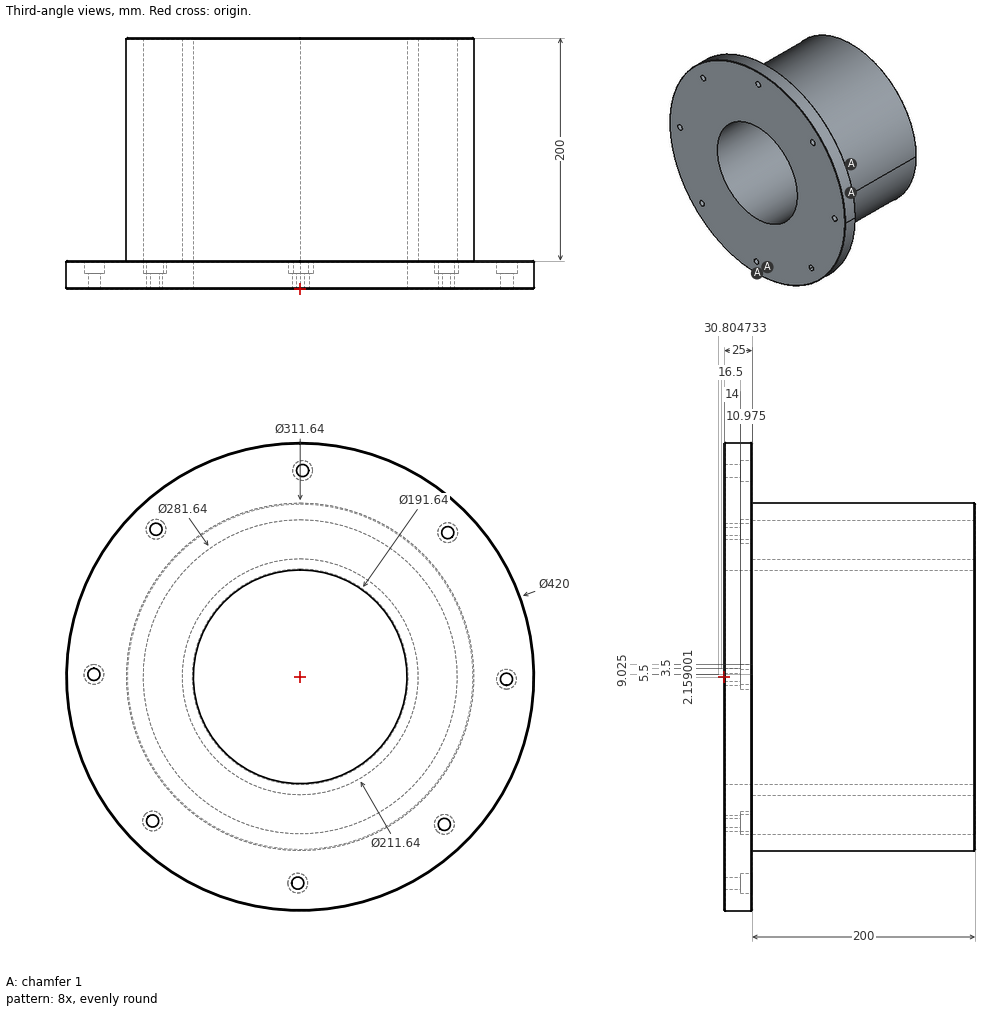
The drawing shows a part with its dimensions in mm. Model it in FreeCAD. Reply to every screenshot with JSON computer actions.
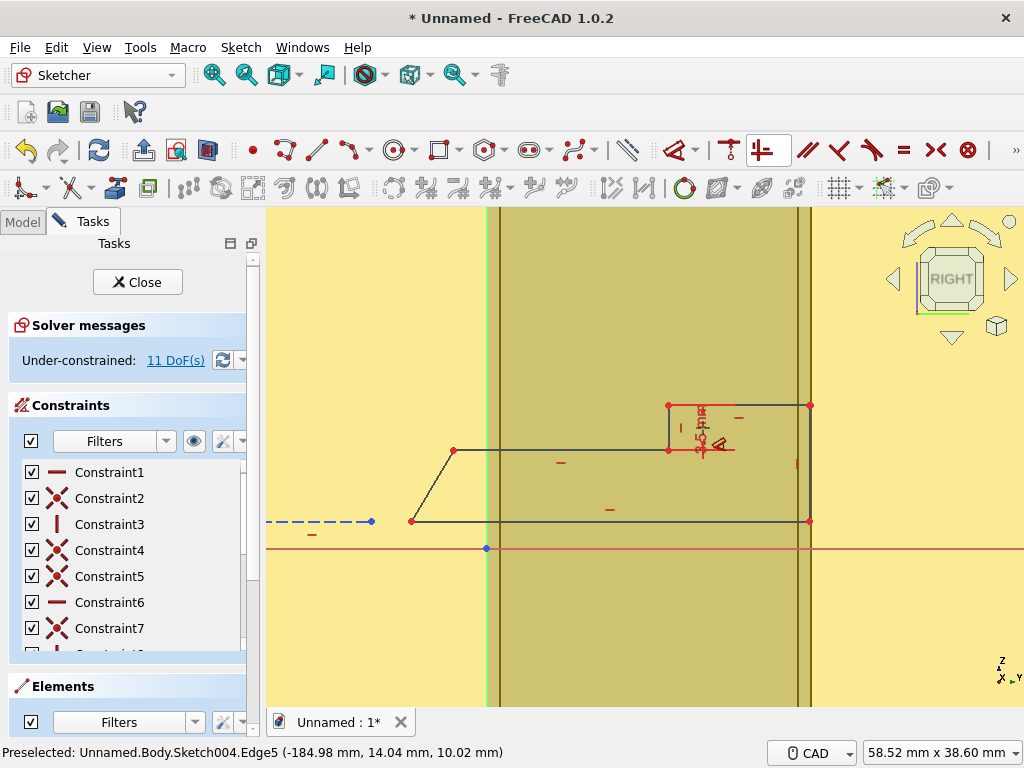
{"action": "left_click", "coordinate": [810, 522]}
{"action": "left_click", "coordinate": [648, 583]}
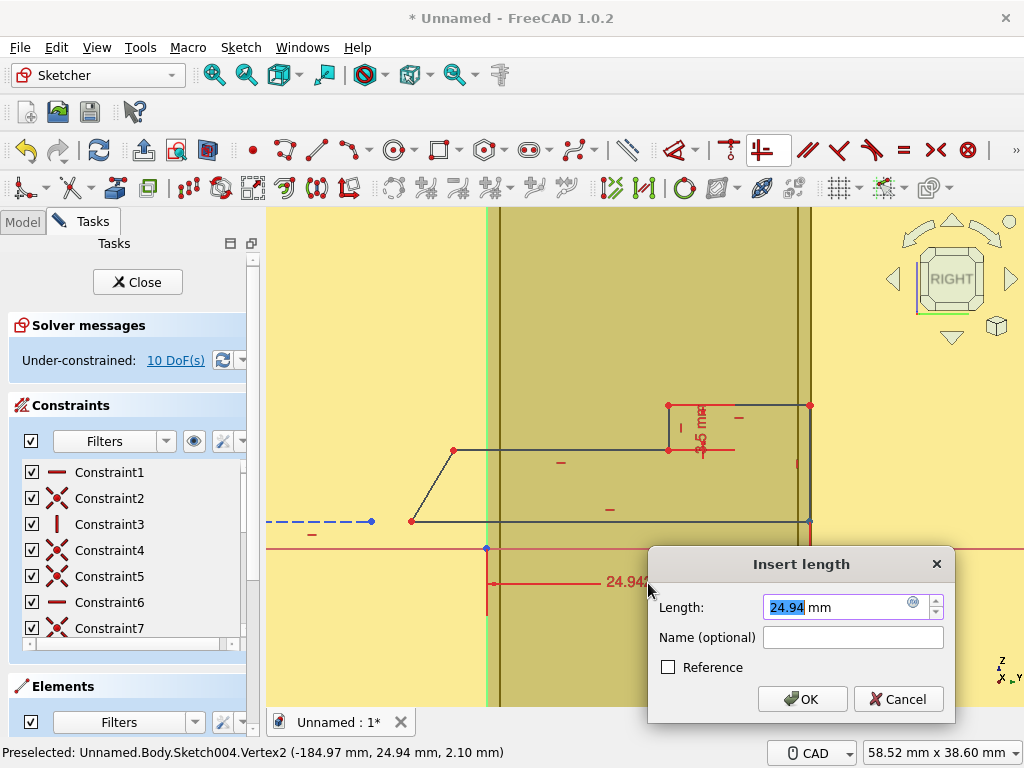
{"action": "type", "text": "25"}
{"action": "key", "text": "Return"}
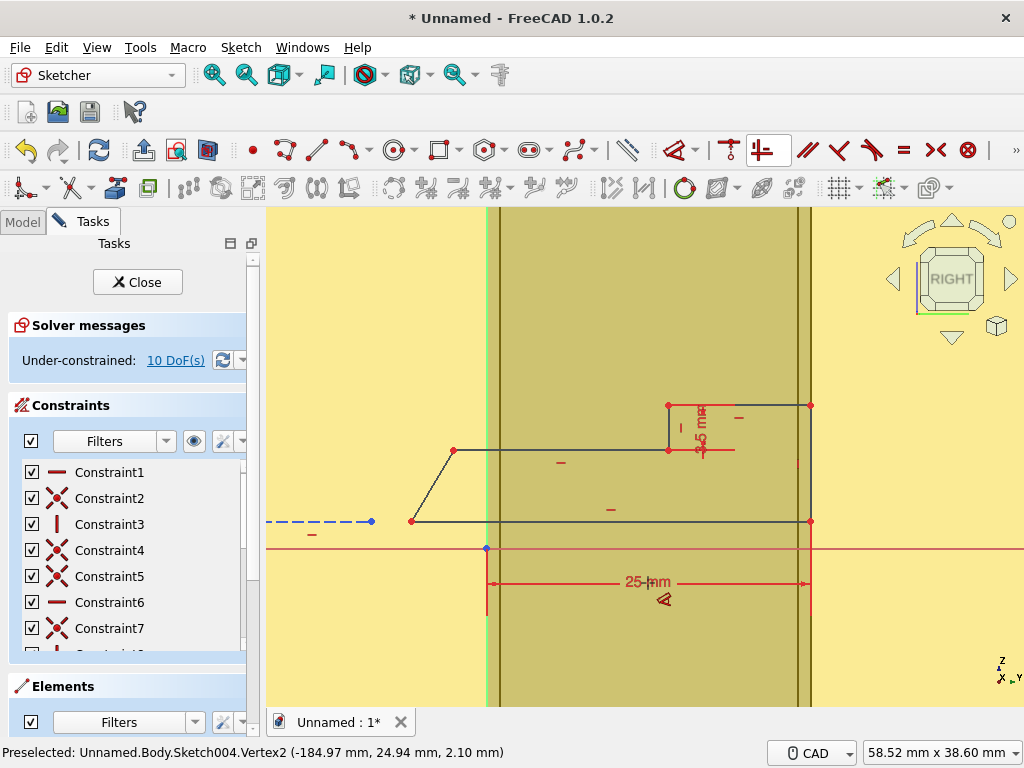
{"action": "left_click", "coordinate": [669, 405]}
{"action": "left_click", "coordinate": [578, 583]}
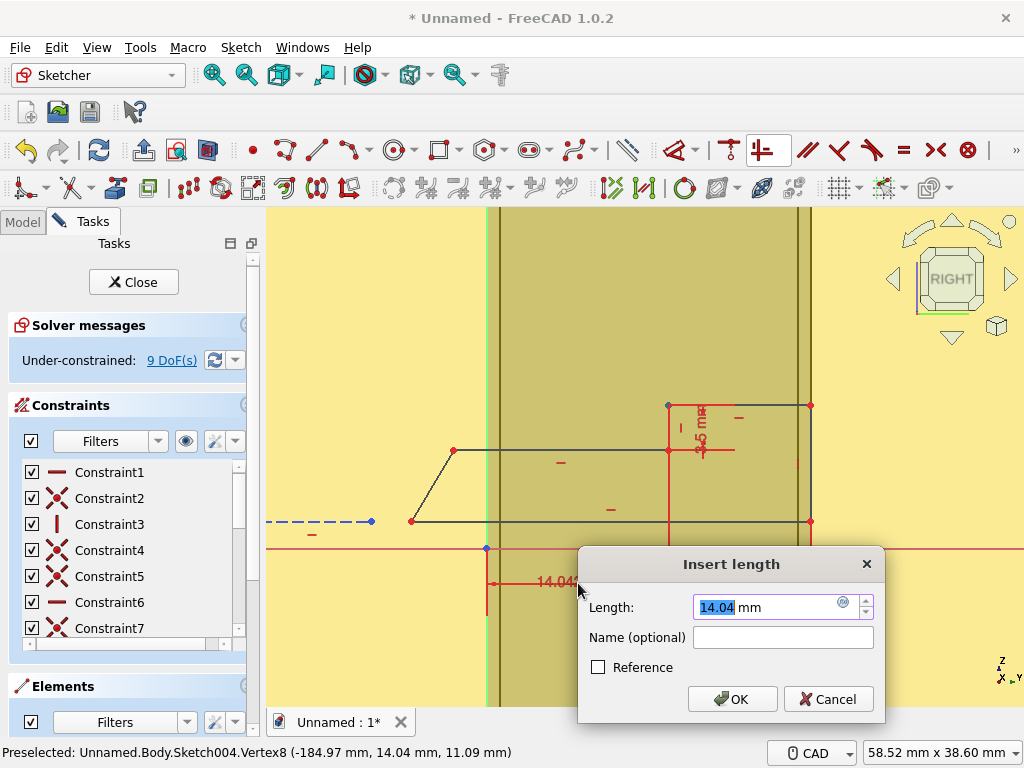
{"action": "type", "text": "14"}
{"action": "key", "text": "Return"}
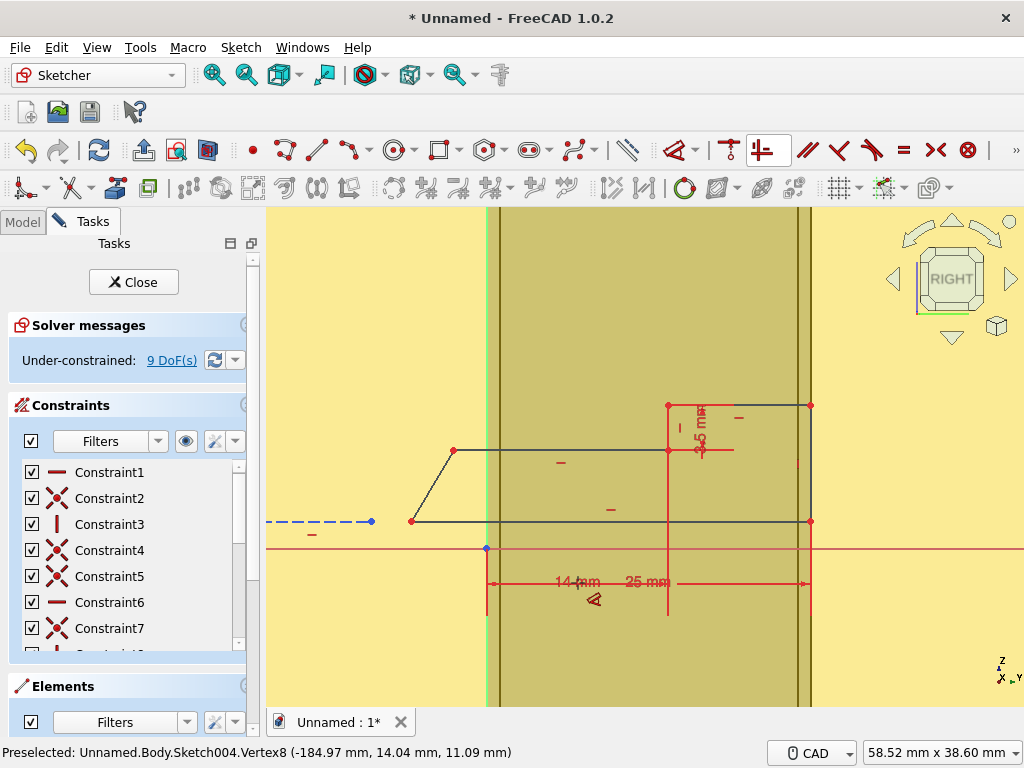
{"action": "left_click", "coordinate": [604, 450]}
{"action": "left_click", "coordinate": [561, 416]}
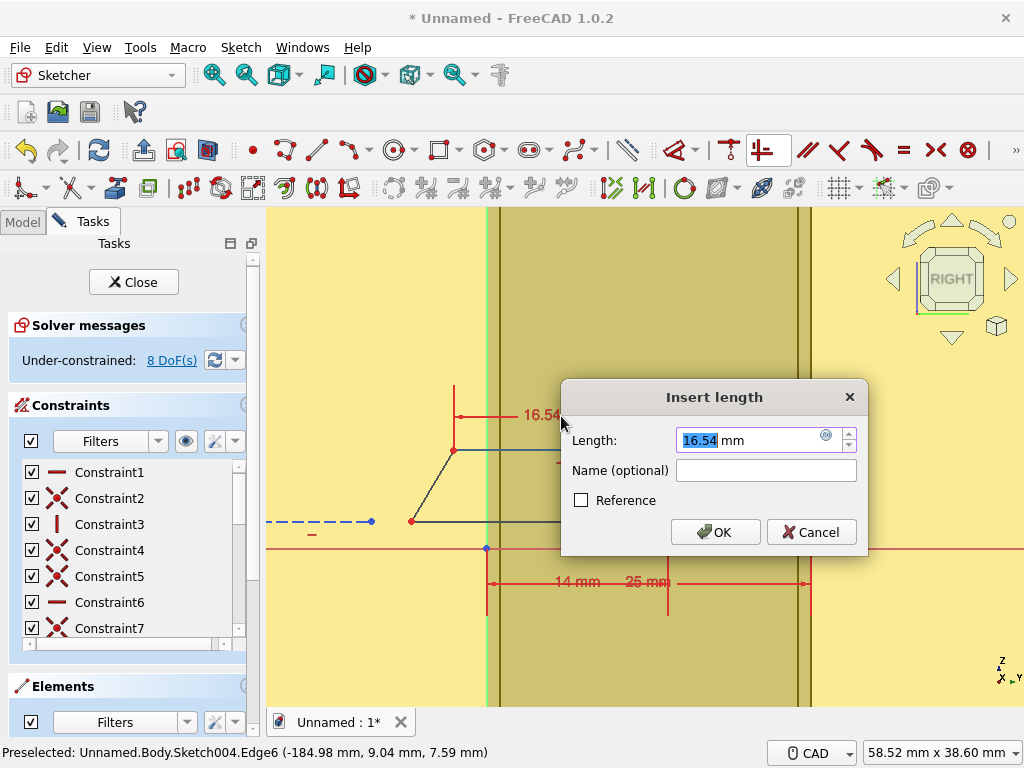
{"action": "type", "text": "16.5"}
{"action": "key", "text": "Return"}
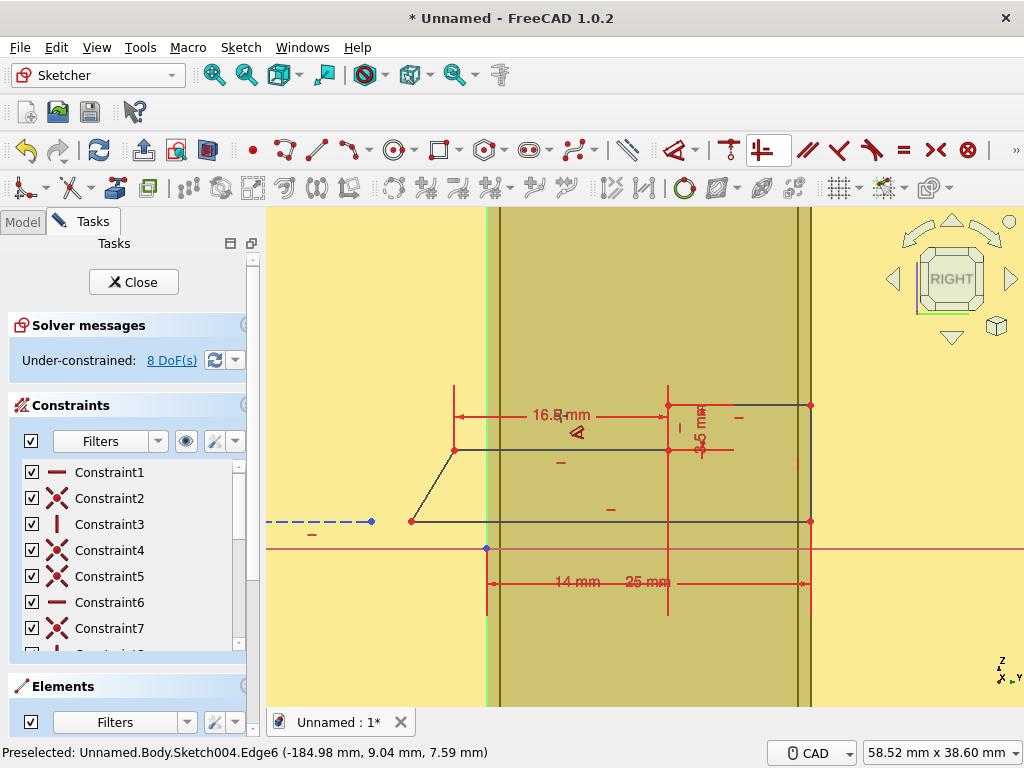
{"action": "left_click", "coordinate": [442, 472]}
{"action": "left_click", "coordinate": [378, 486]}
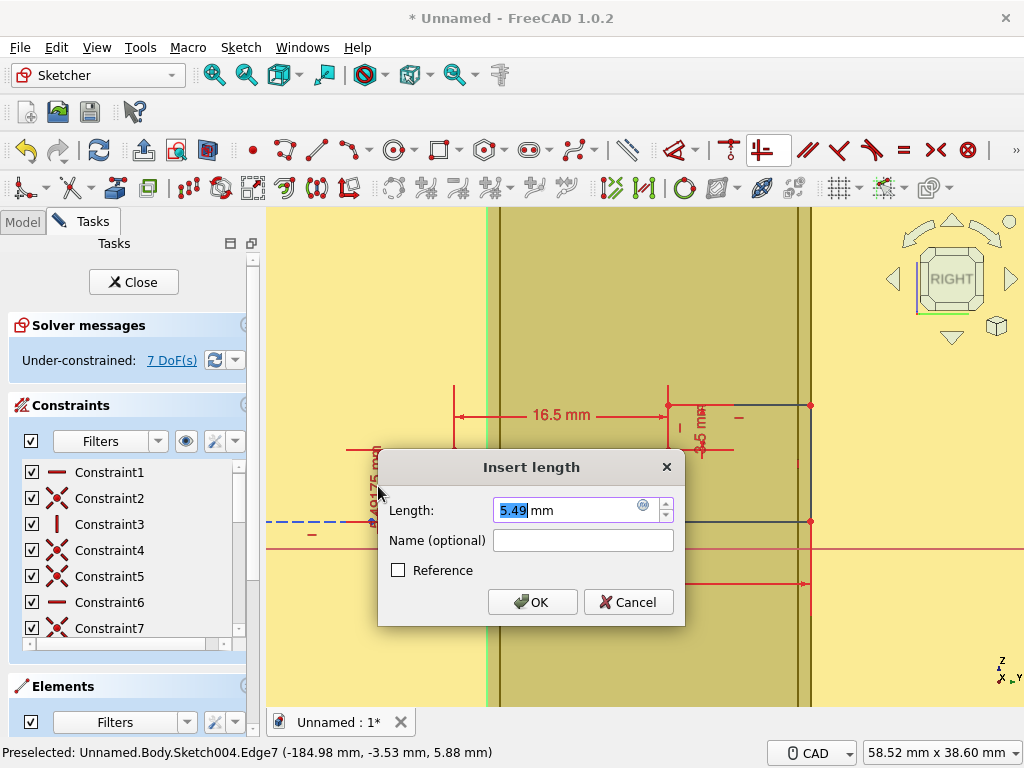
{"action": "type", "text": "5.5"}
{"action": "key", "text": "Return"}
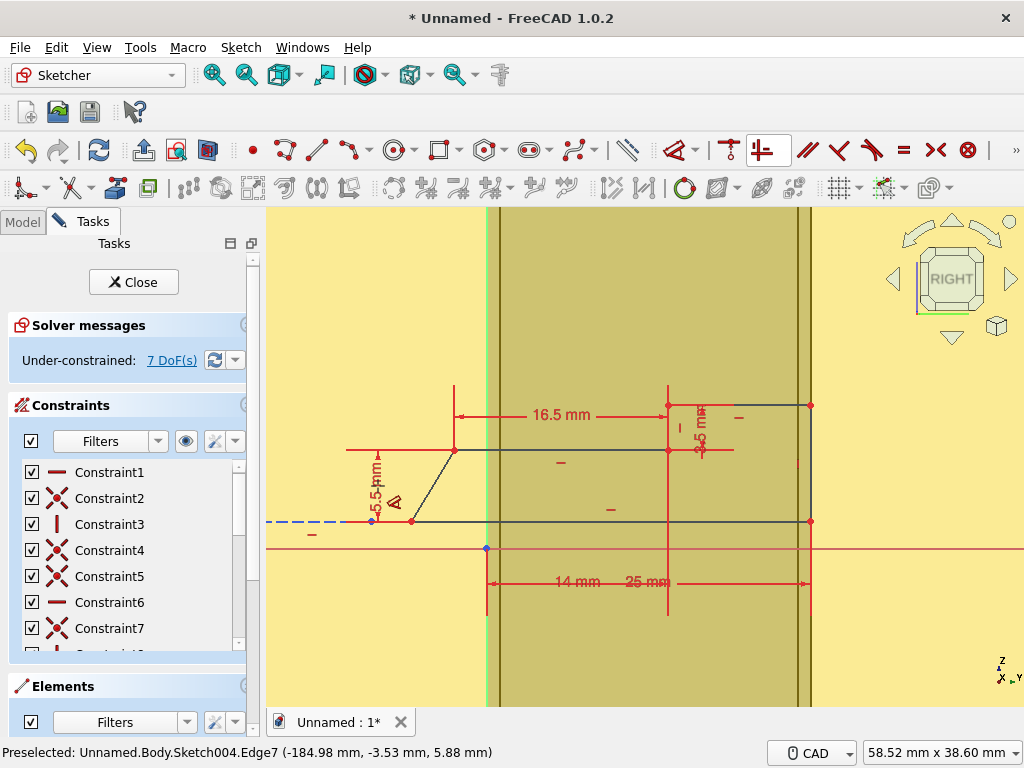
{"action": "left_click", "coordinate": [811, 487]}
{"action": "left_click", "coordinate": [845, 463]}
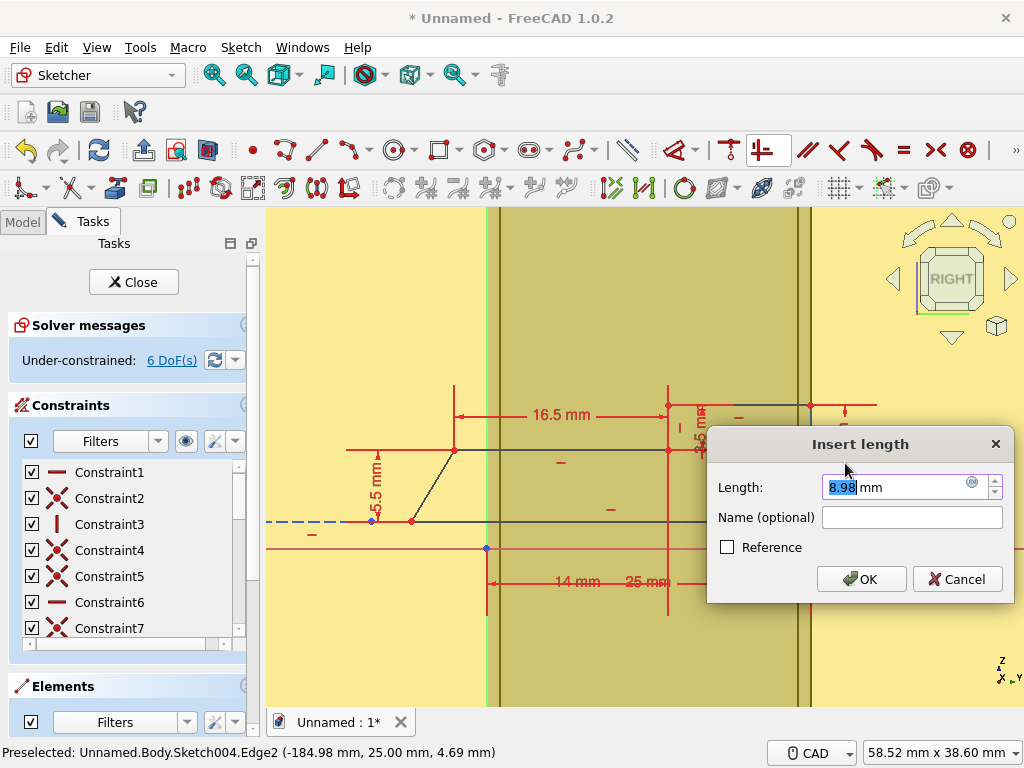
{"action": "type", "text": "9.025"}
{"action": "key", "text": "Return"}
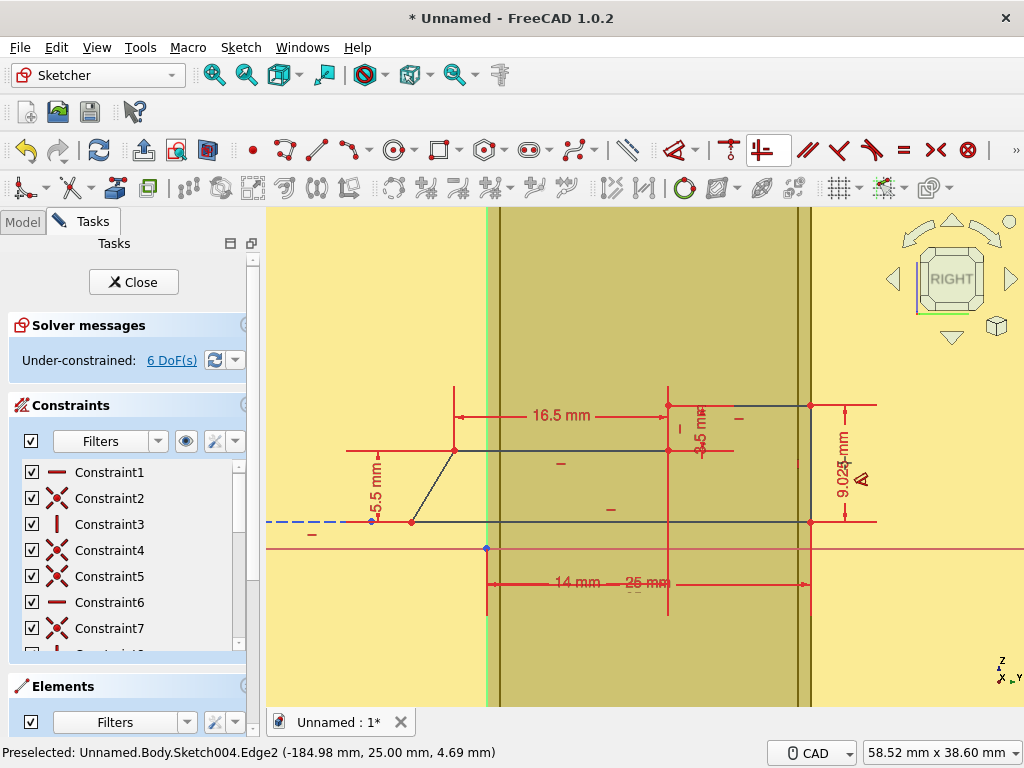
{"action": "left_click", "coordinate": [768, 406]}
{"action": "left_click", "coordinate": [739, 372]}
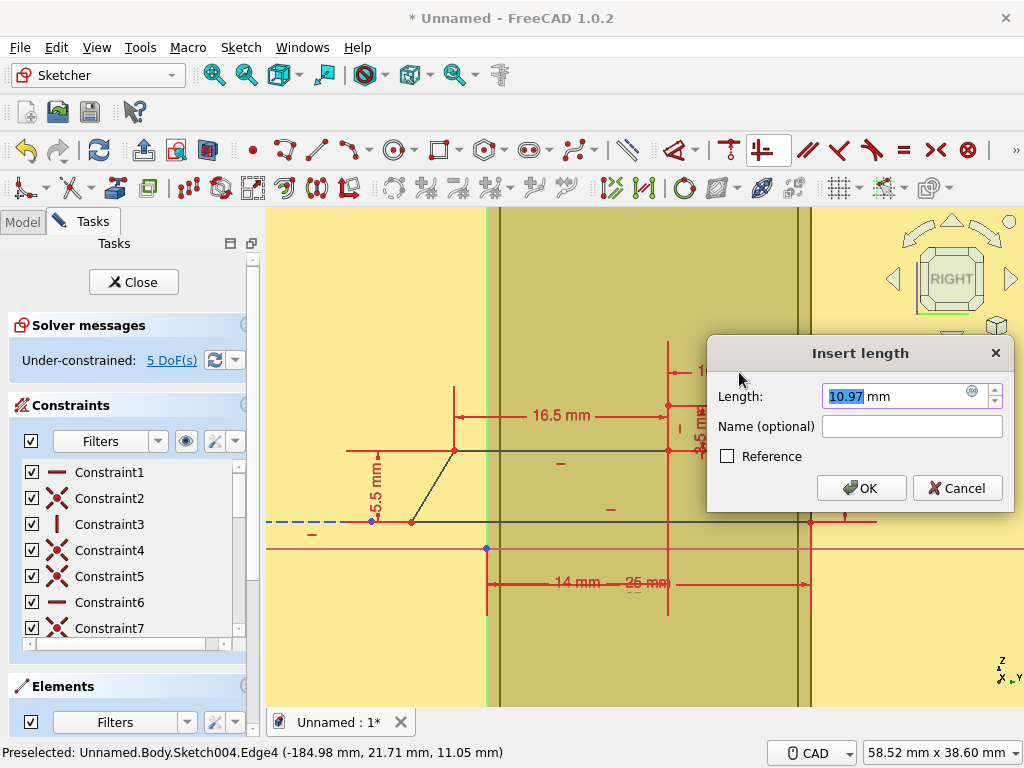
{"action": "type", "text": "10.975"}
{"action": "key", "text": "Return"}